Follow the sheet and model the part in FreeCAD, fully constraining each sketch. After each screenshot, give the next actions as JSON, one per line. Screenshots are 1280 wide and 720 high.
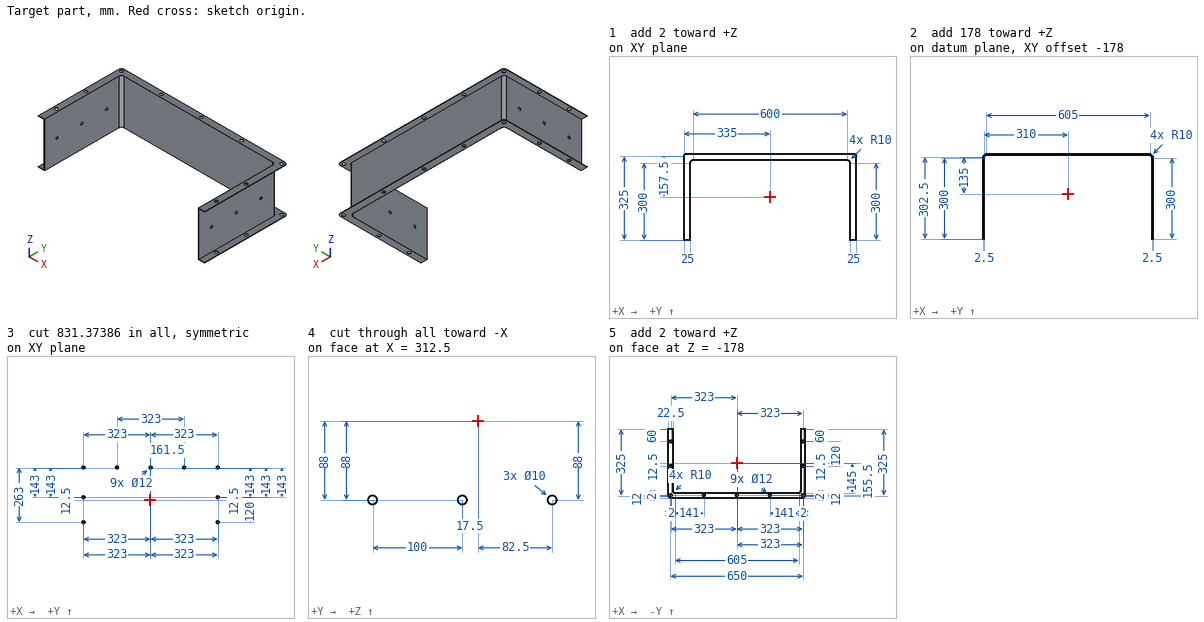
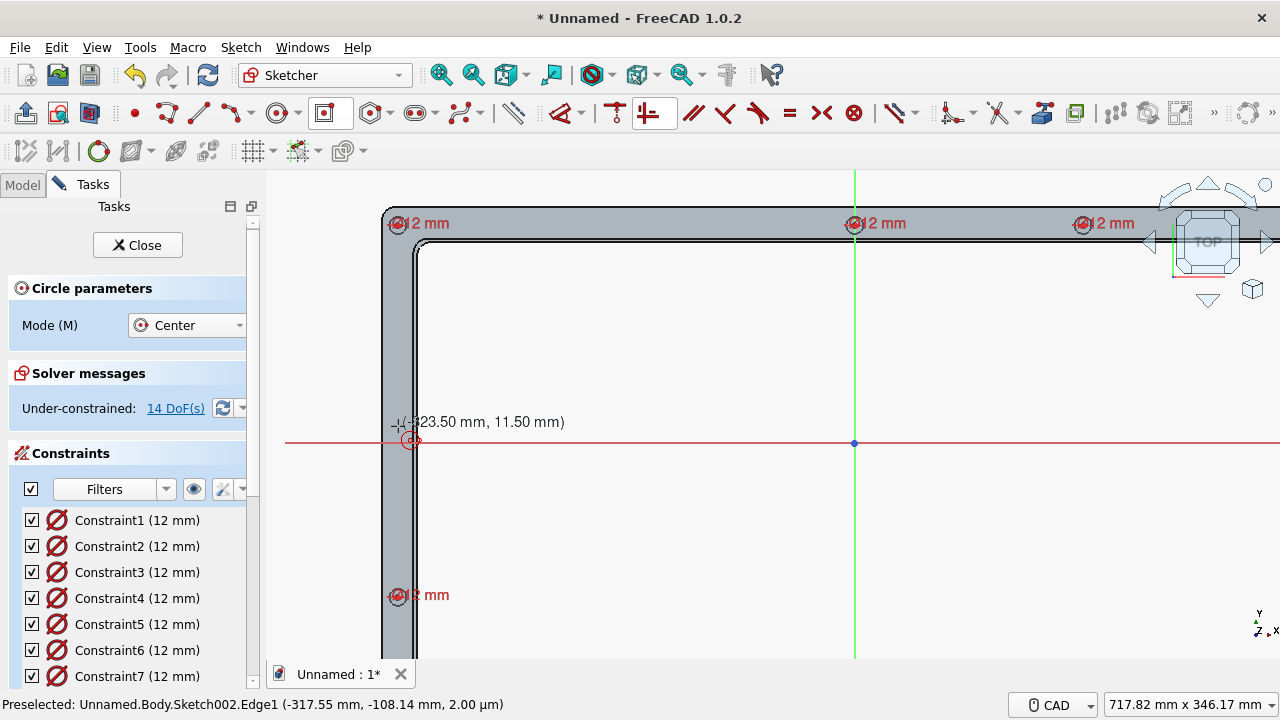
{"action": "left_click", "coordinate": [399, 426]}
{"action": "mouse_move", "coordinate": [405, 420]}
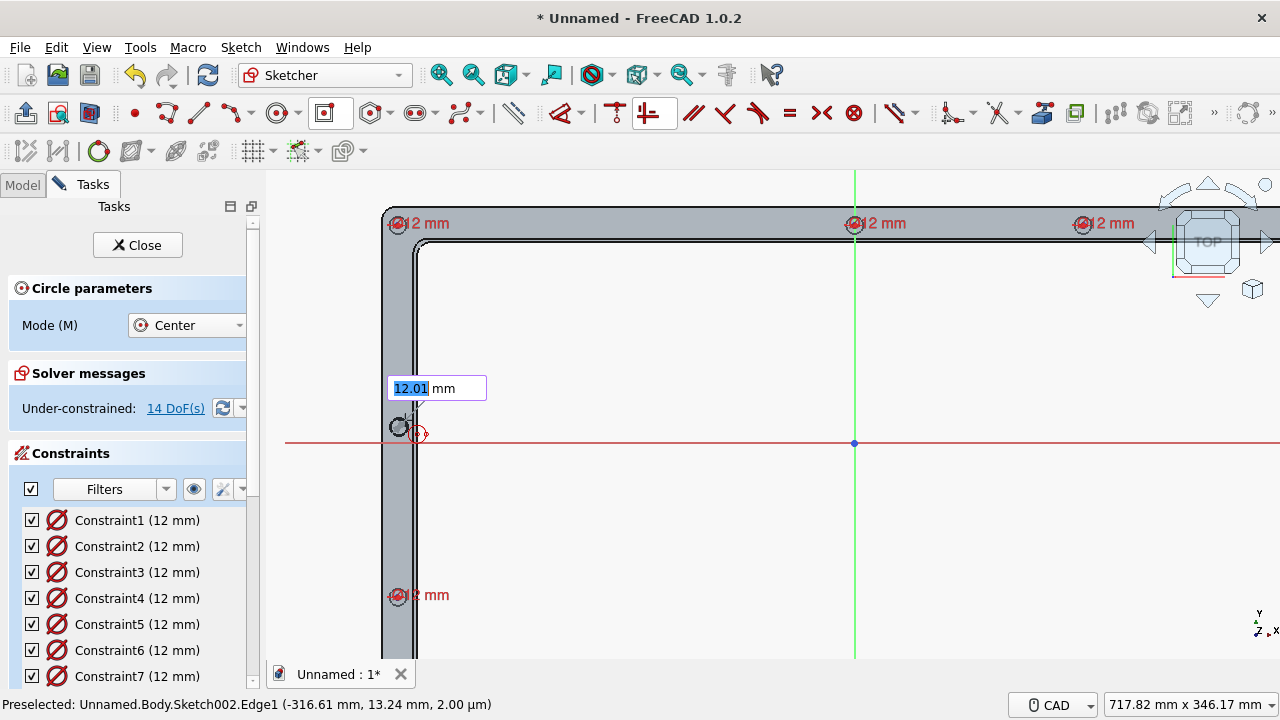
{"action": "type", "text": "12"}
{"action": "key", "text": "Return"}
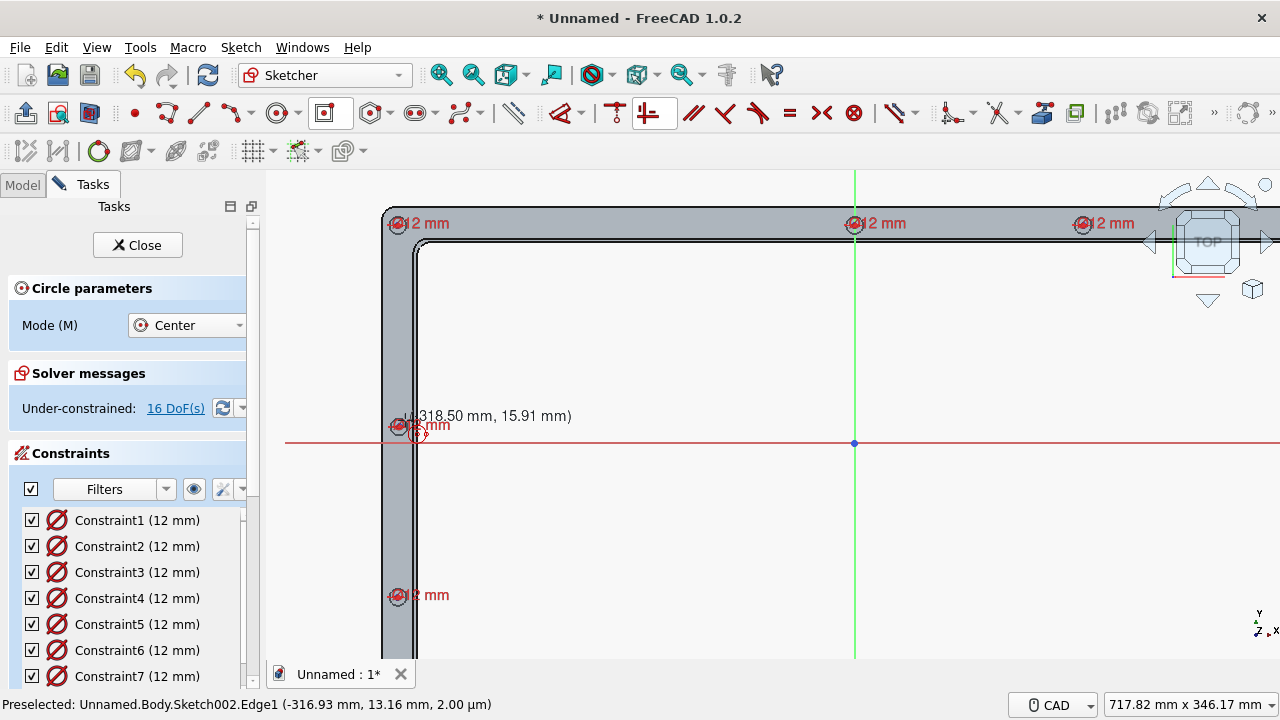
{"action": "scroll", "coordinate": [627, 224], "scroll_direction": "up", "scroll_amount": 5}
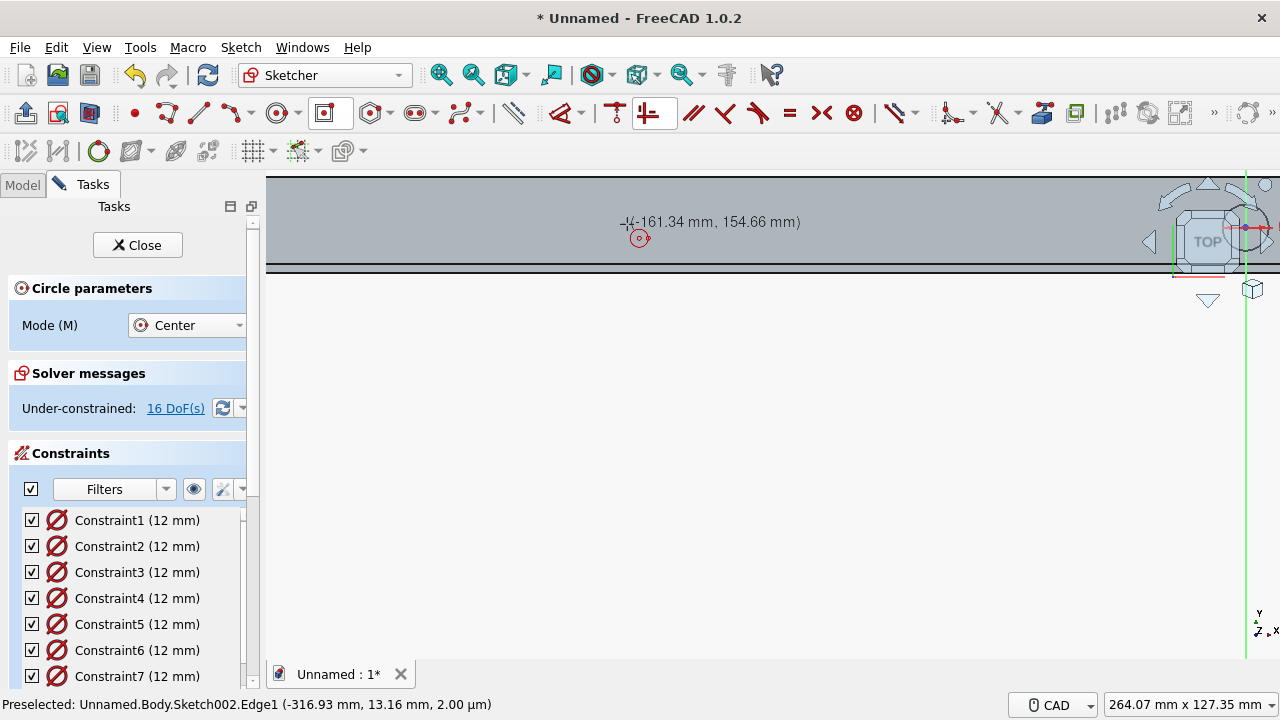
{"action": "scroll", "coordinate": [527, 312], "scroll_direction": "down", "scroll_amount": 7}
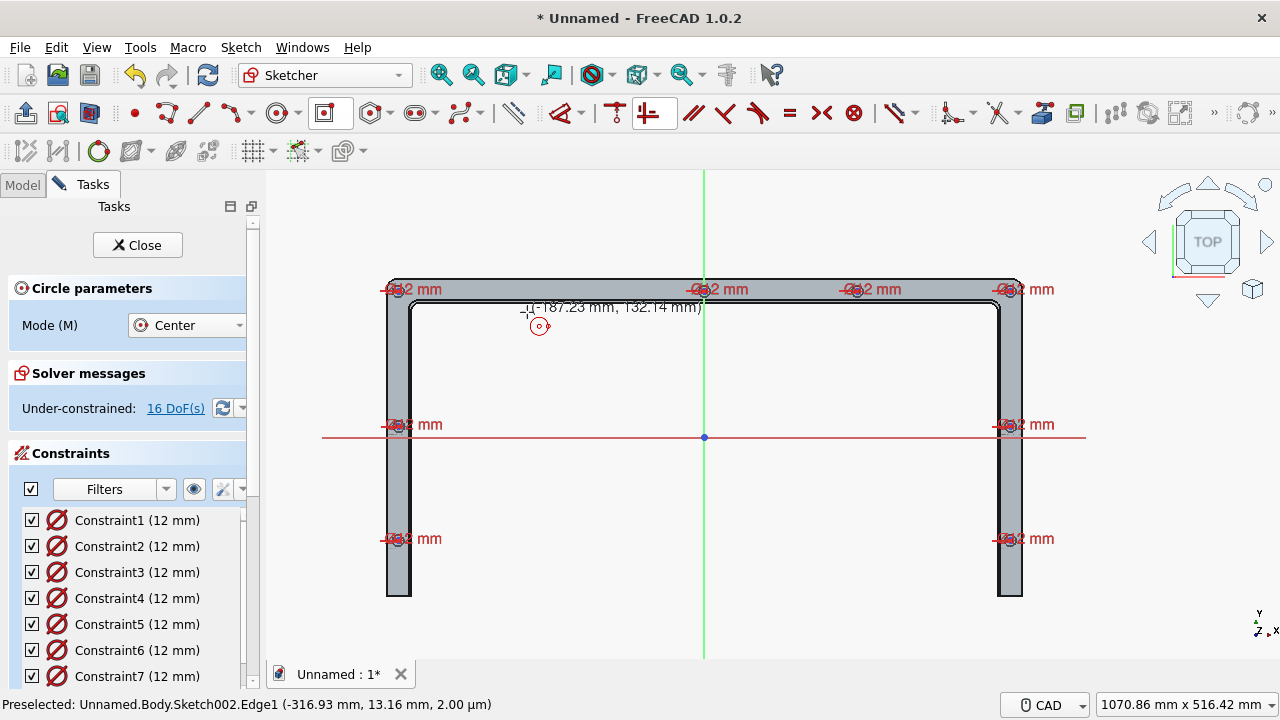
{"action": "left_click", "coordinate": [552, 290]}
{"action": "mouse_move", "coordinate": [556, 286]}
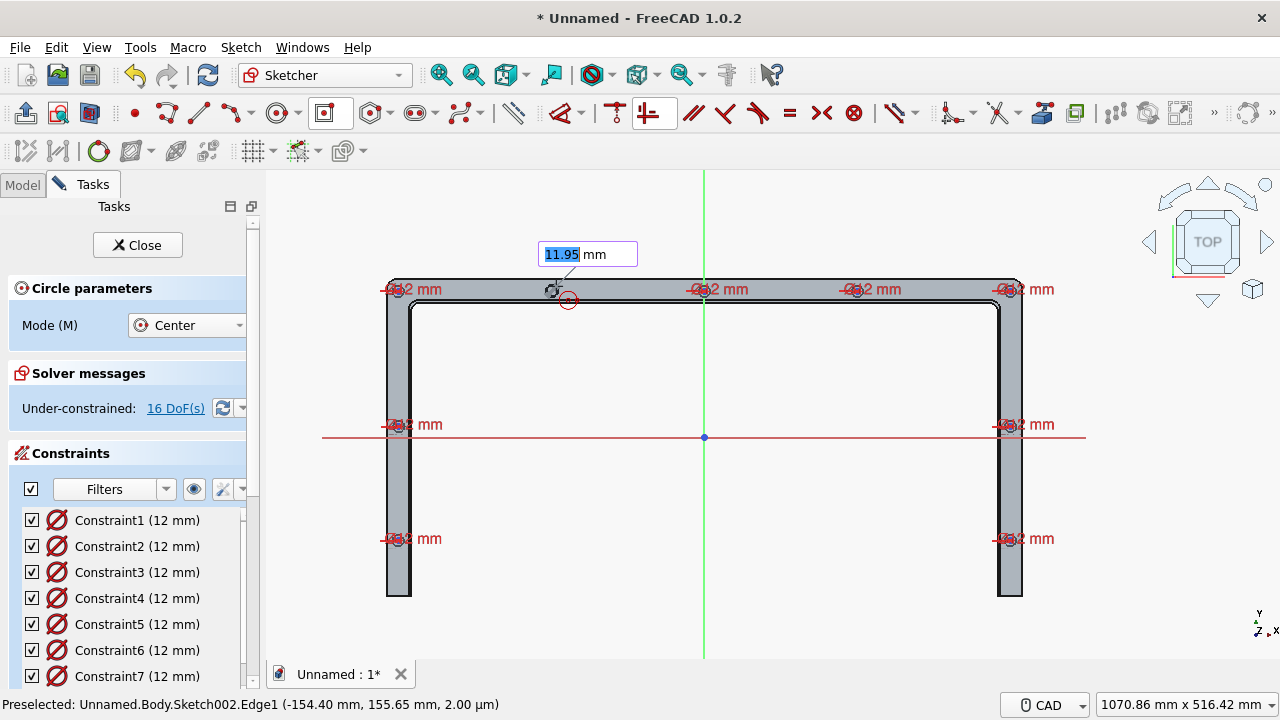
{"action": "type", "text": "12"}
{"action": "key", "text": "Return"}
{"action": "key", "text": "Escape"}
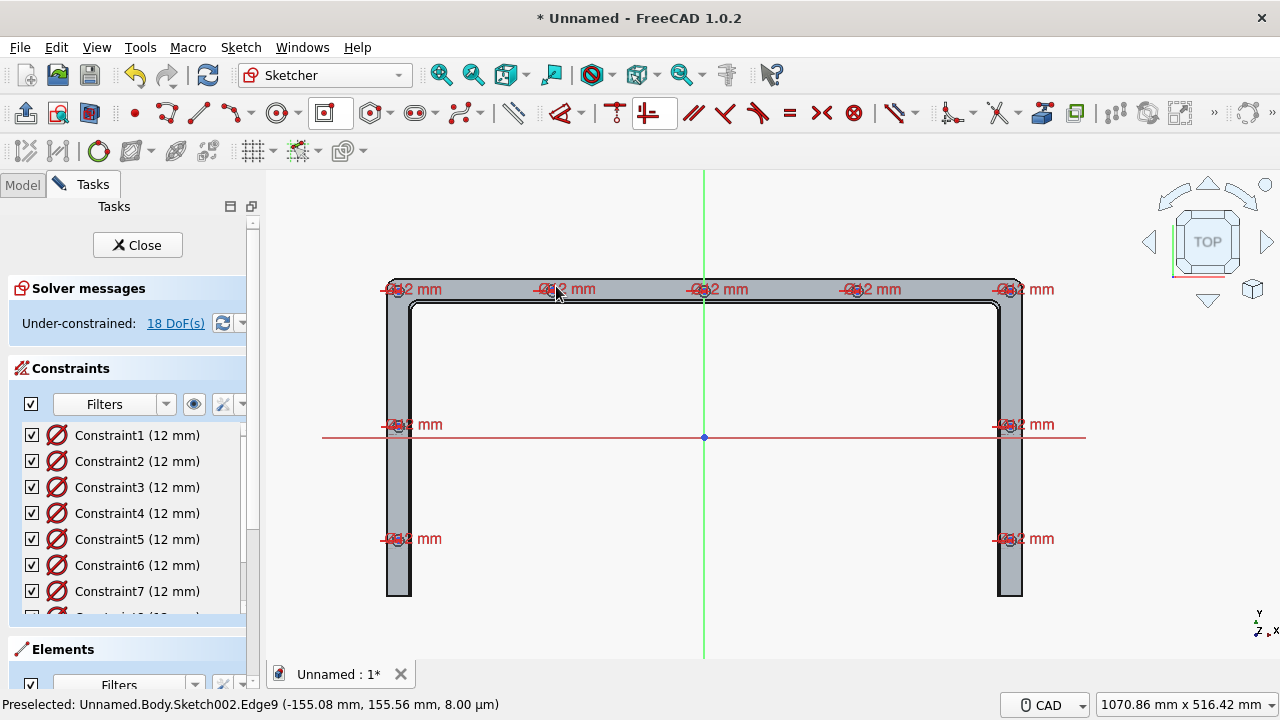
{"action": "left_click", "coordinate": [704, 291]}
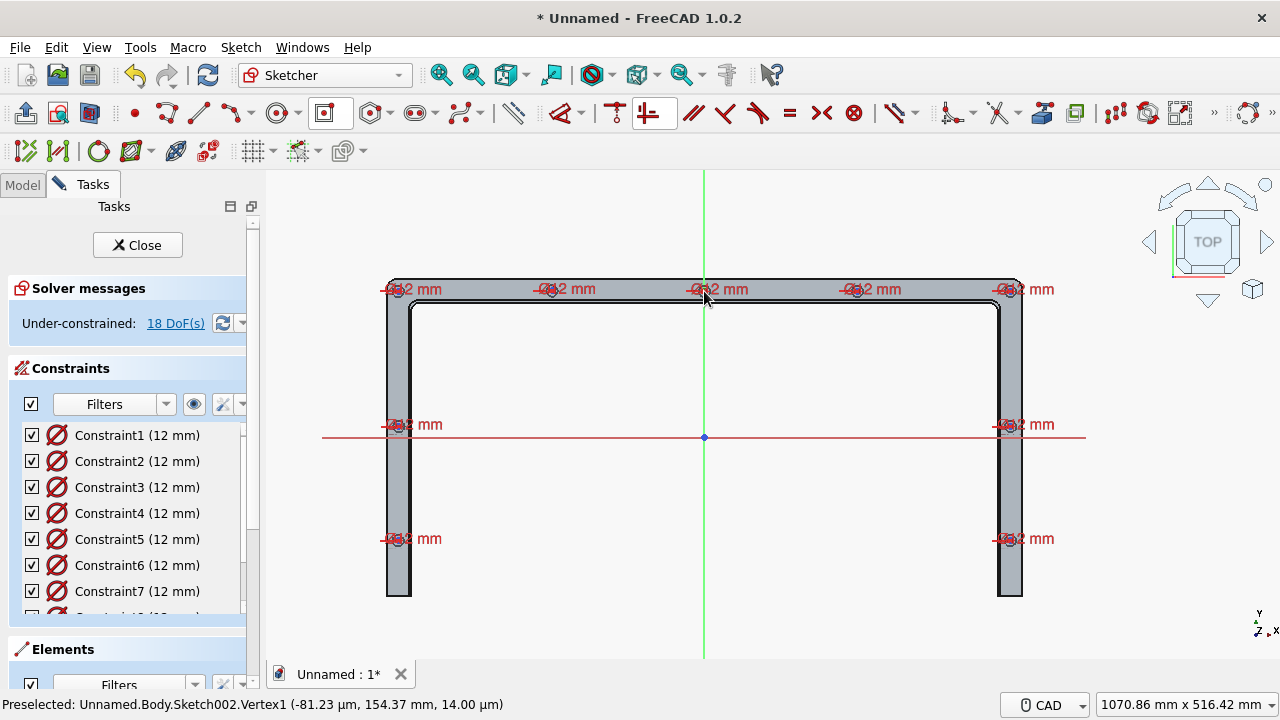
{"action": "left_click", "coordinate": [704, 600]}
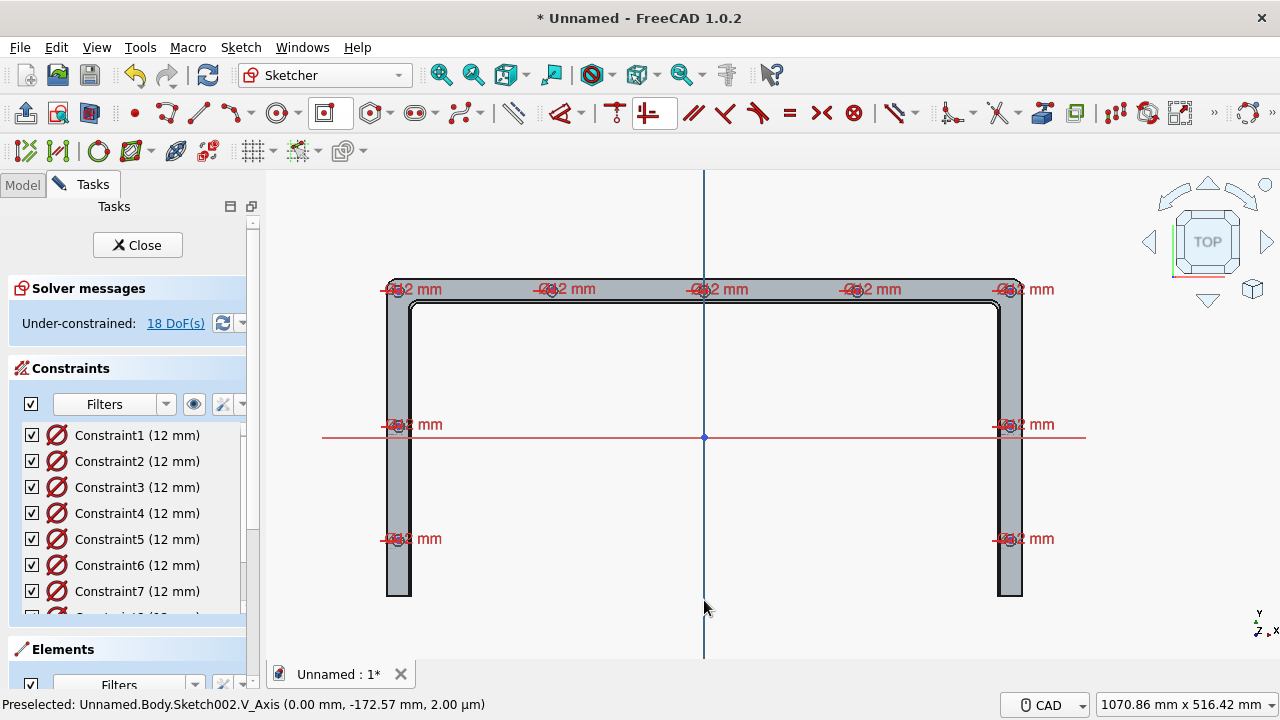
{"action": "left_click", "coordinate": [616, 114]}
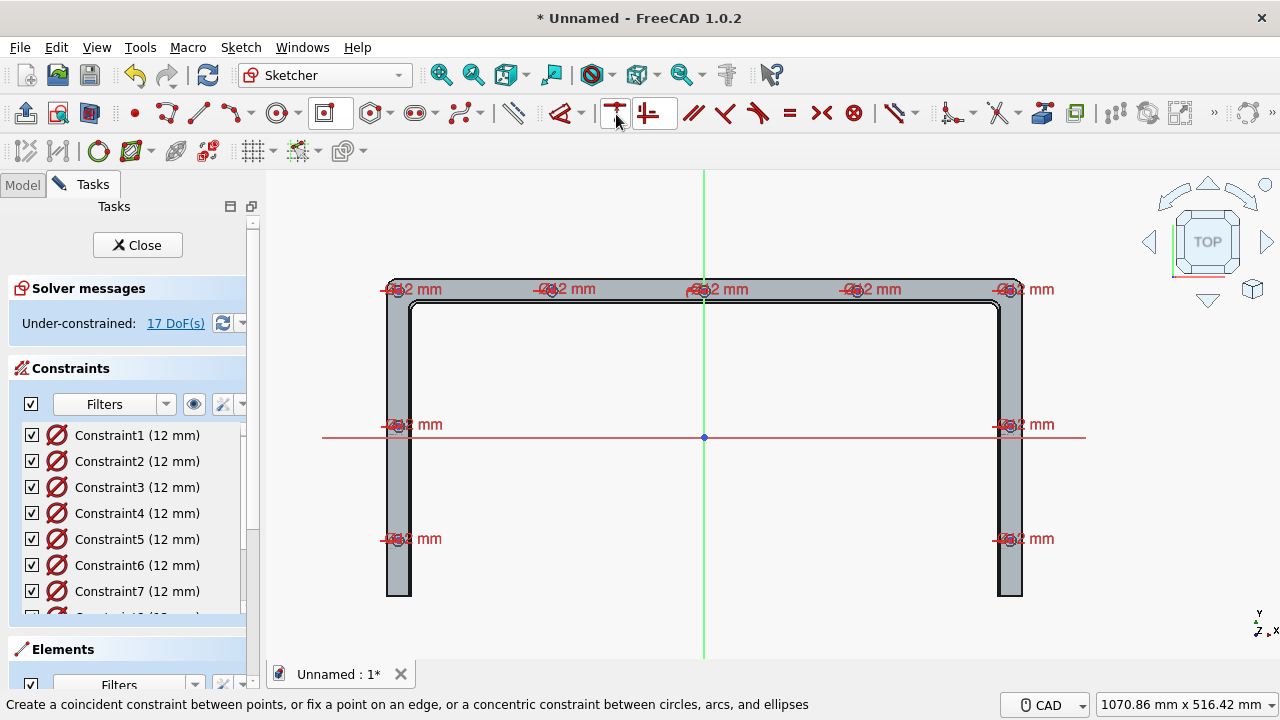
{"action": "left_click", "coordinate": [560, 114]}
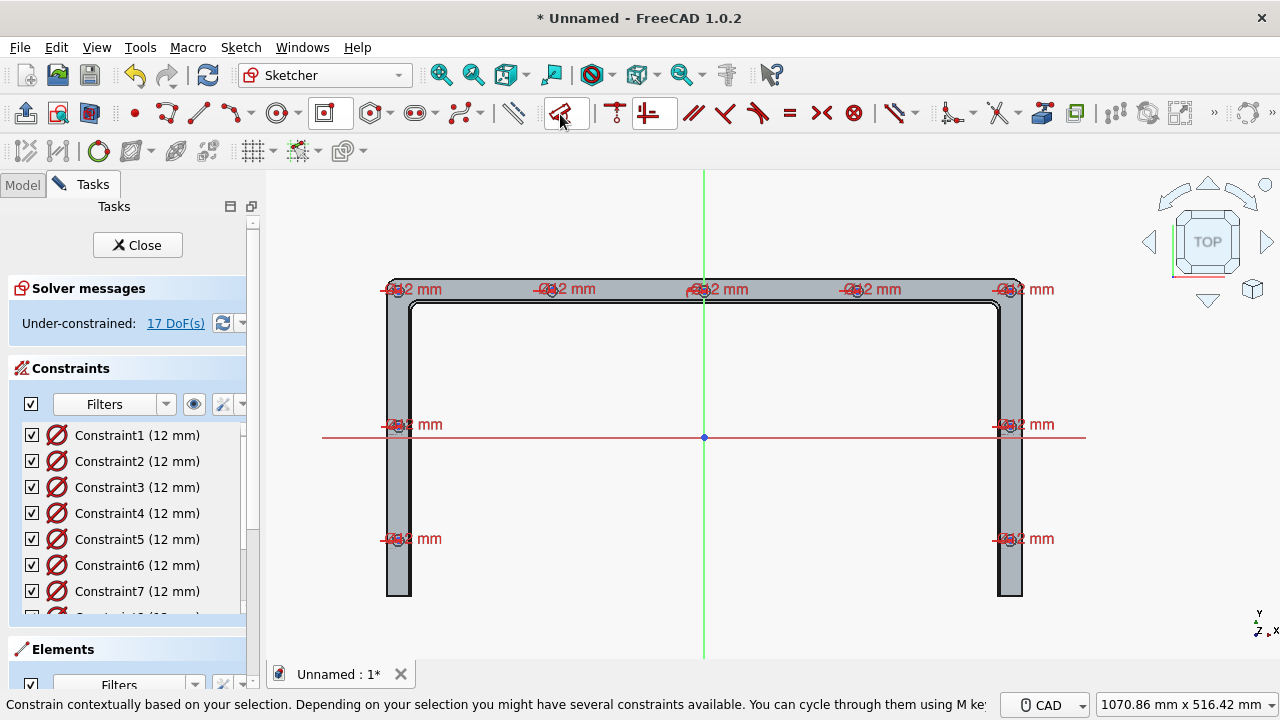
{"action": "left_click", "coordinate": [1011, 427]}
{"action": "left_click", "coordinate": [858, 472]}